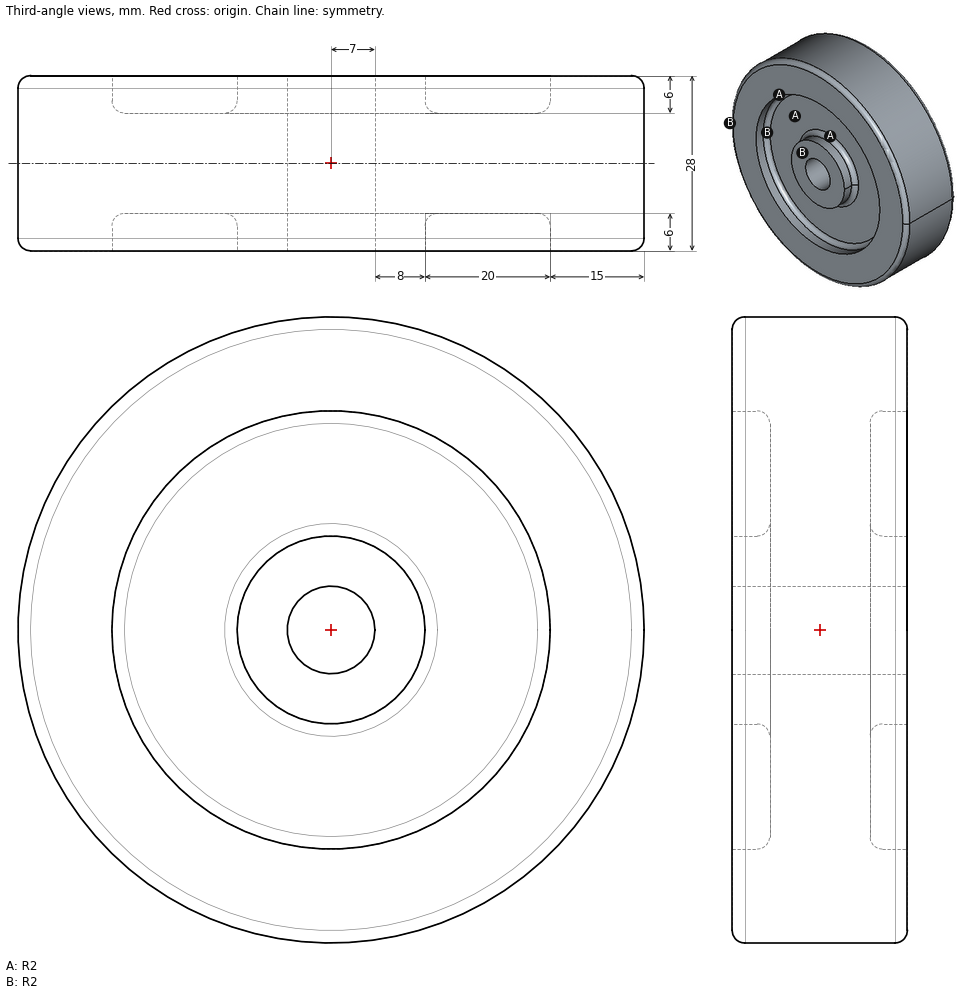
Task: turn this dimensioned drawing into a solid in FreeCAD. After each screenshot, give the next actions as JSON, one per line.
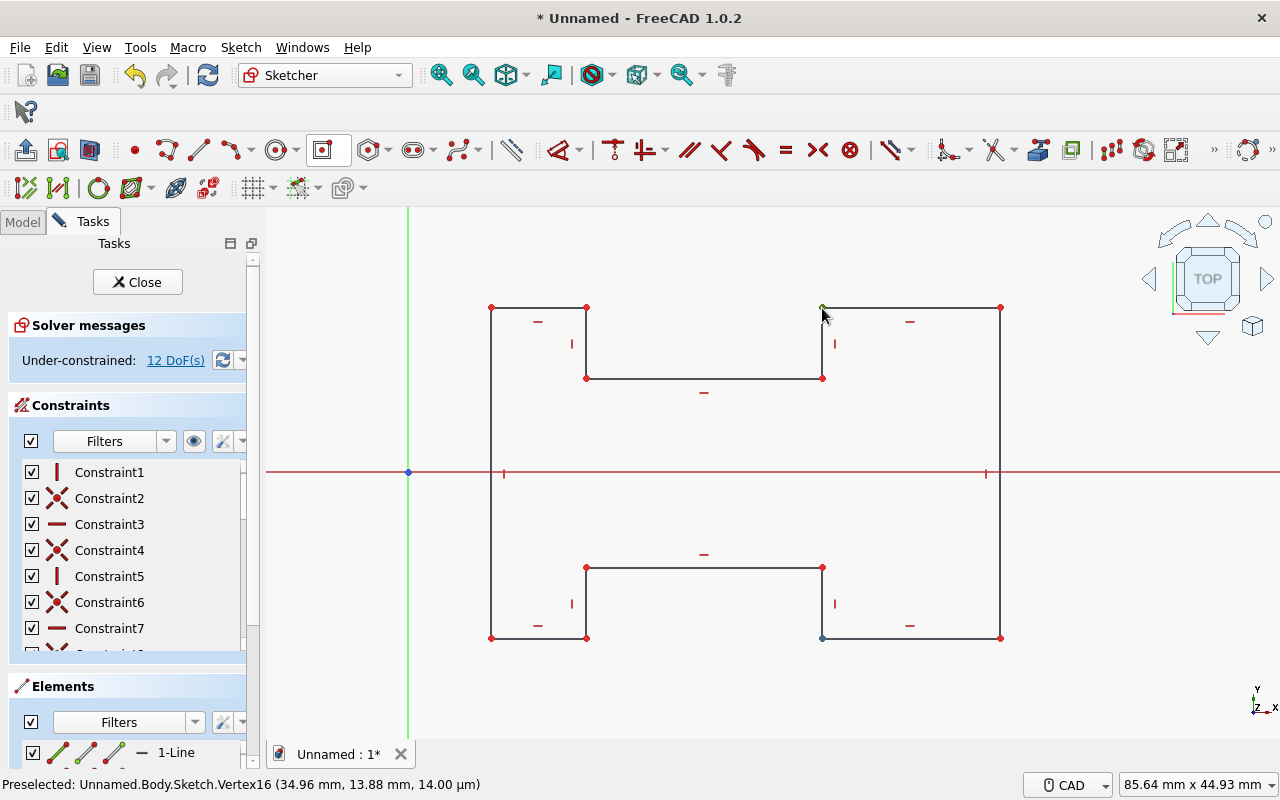
{"action": "left_click", "coordinate": [353, 472]}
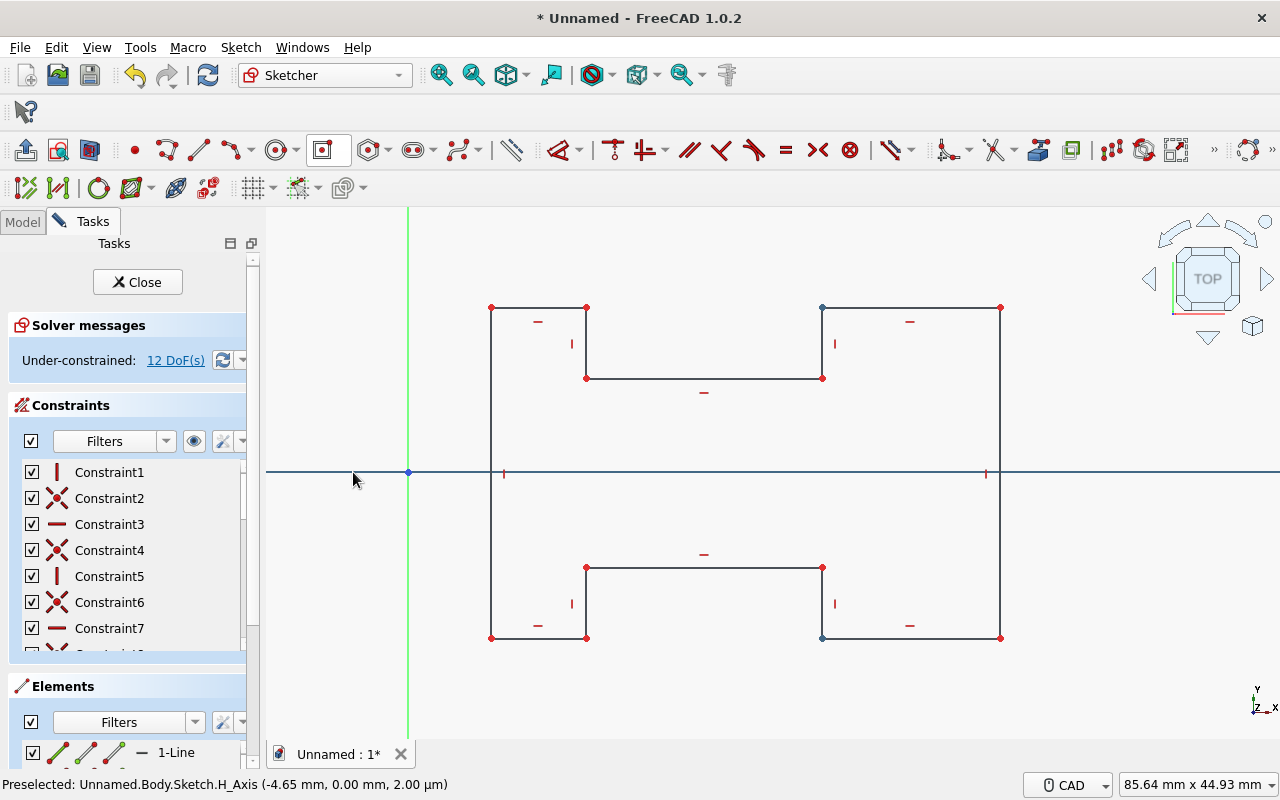
{"action": "left_click", "coordinate": [818, 150]}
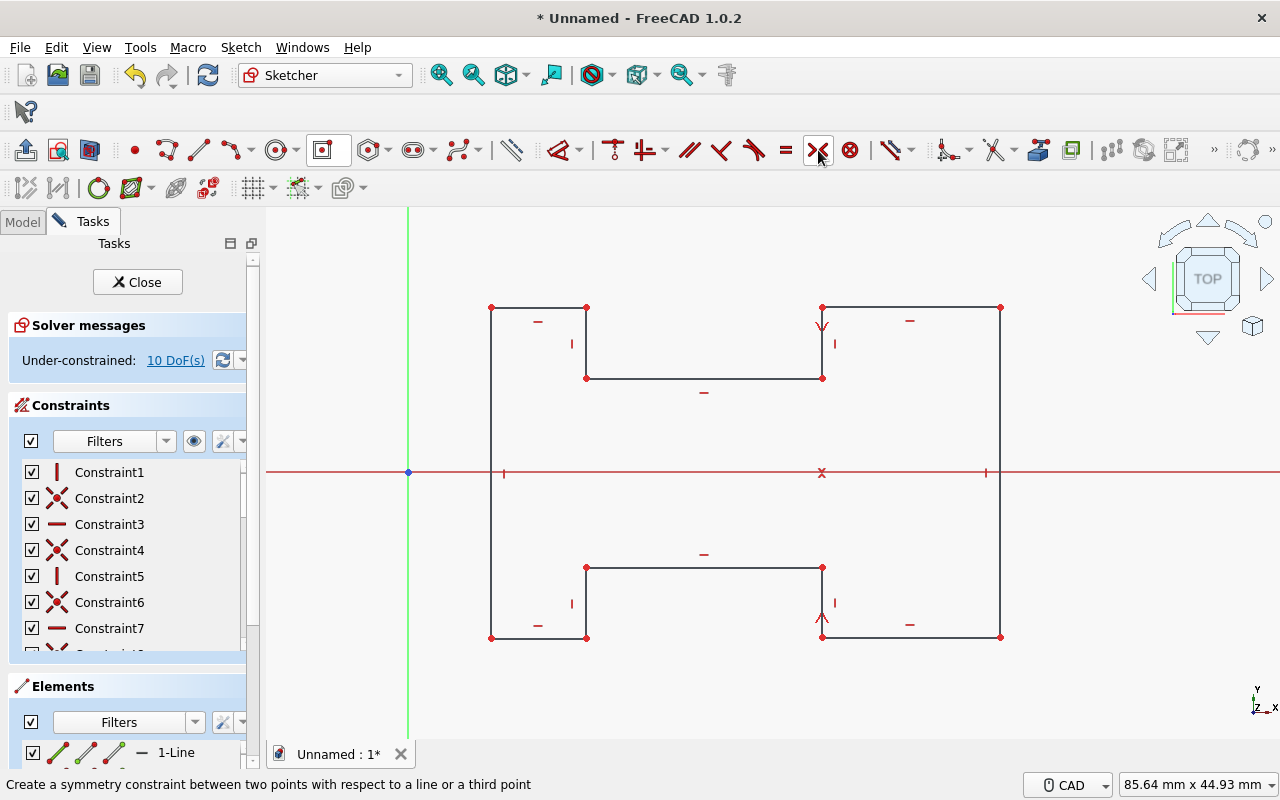
{"action": "left_click", "coordinate": [586, 568]}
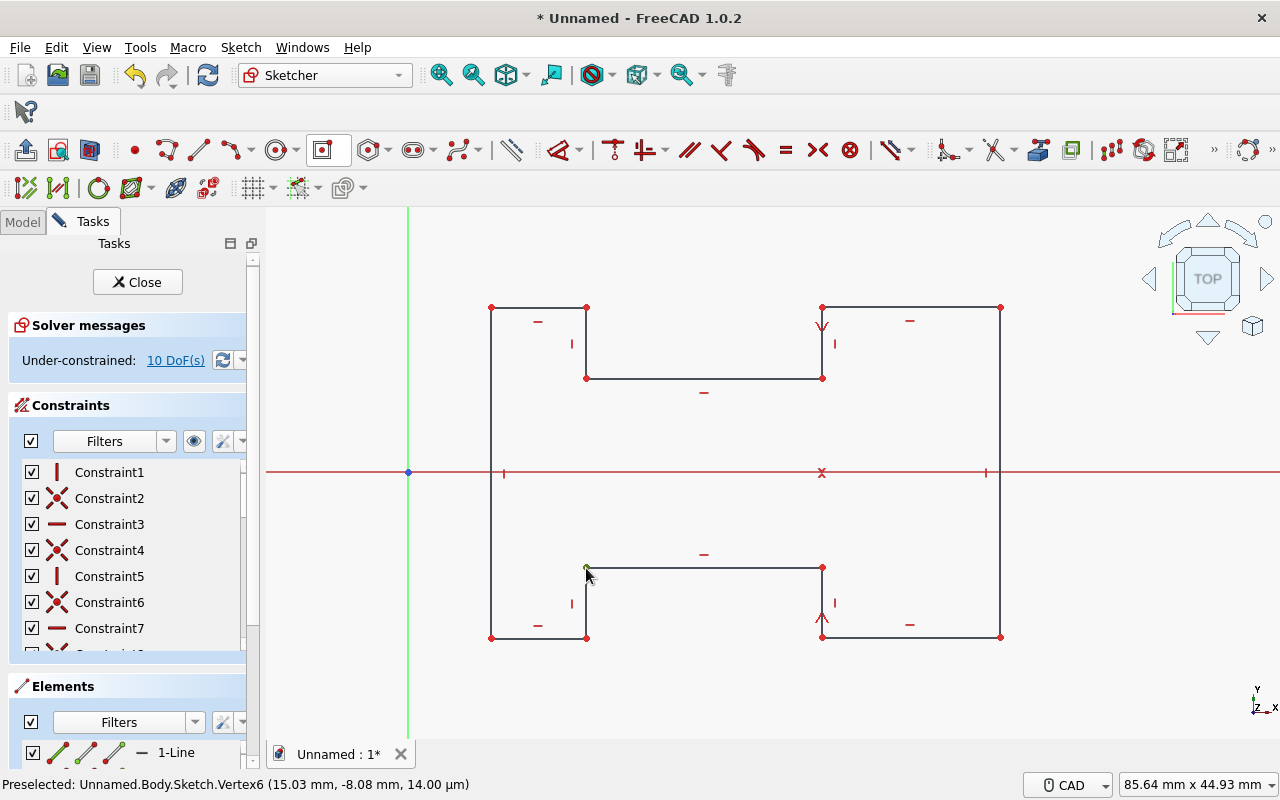
{"action": "left_click", "coordinate": [586, 379]}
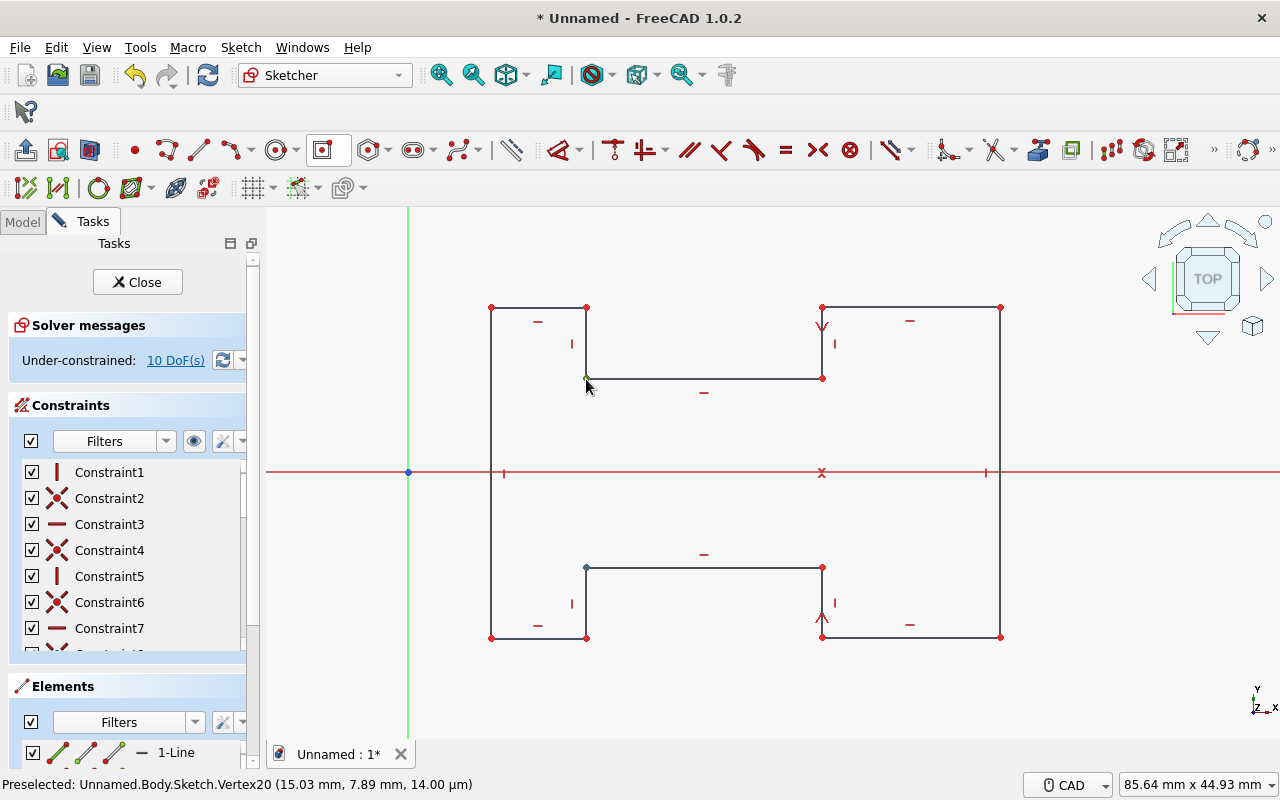
{"action": "left_click", "coordinate": [353, 472]}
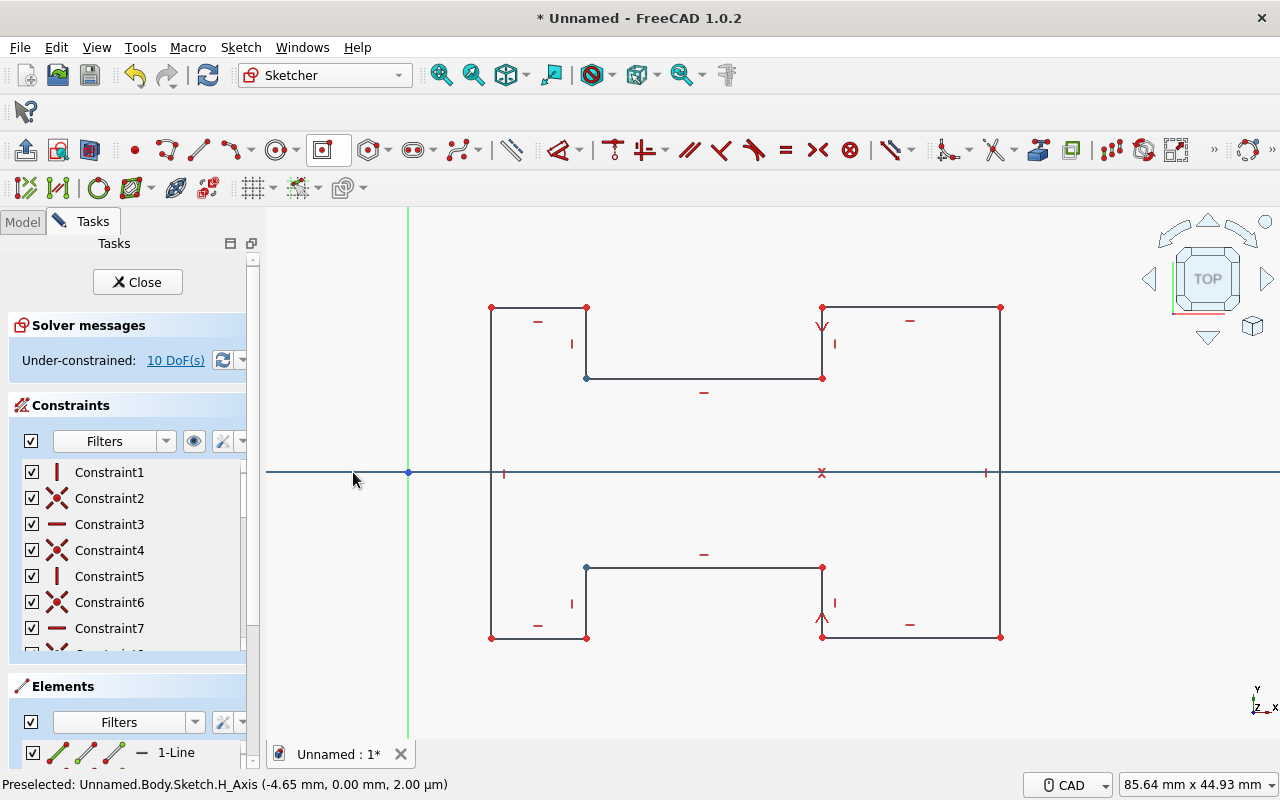
{"action": "left_click", "coordinate": [818, 150]}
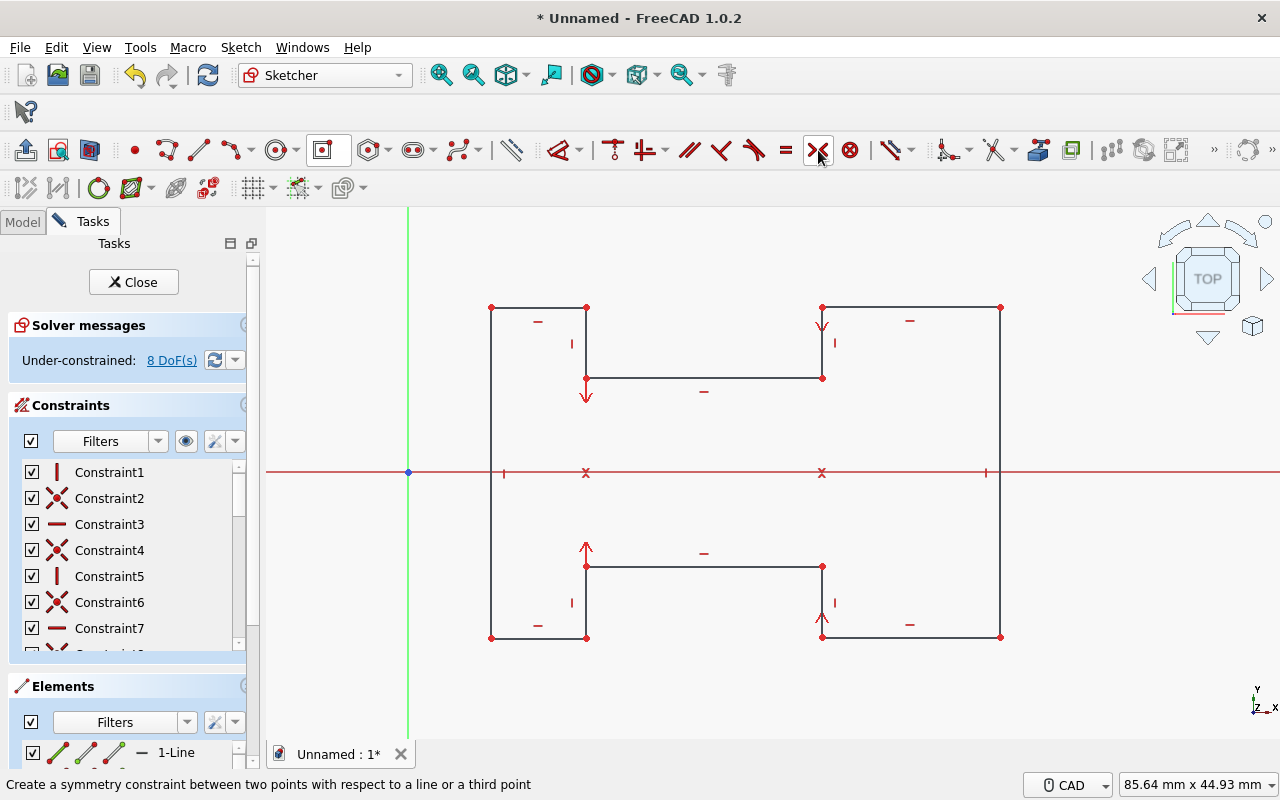
{"action": "left_click", "coordinate": [558, 150]}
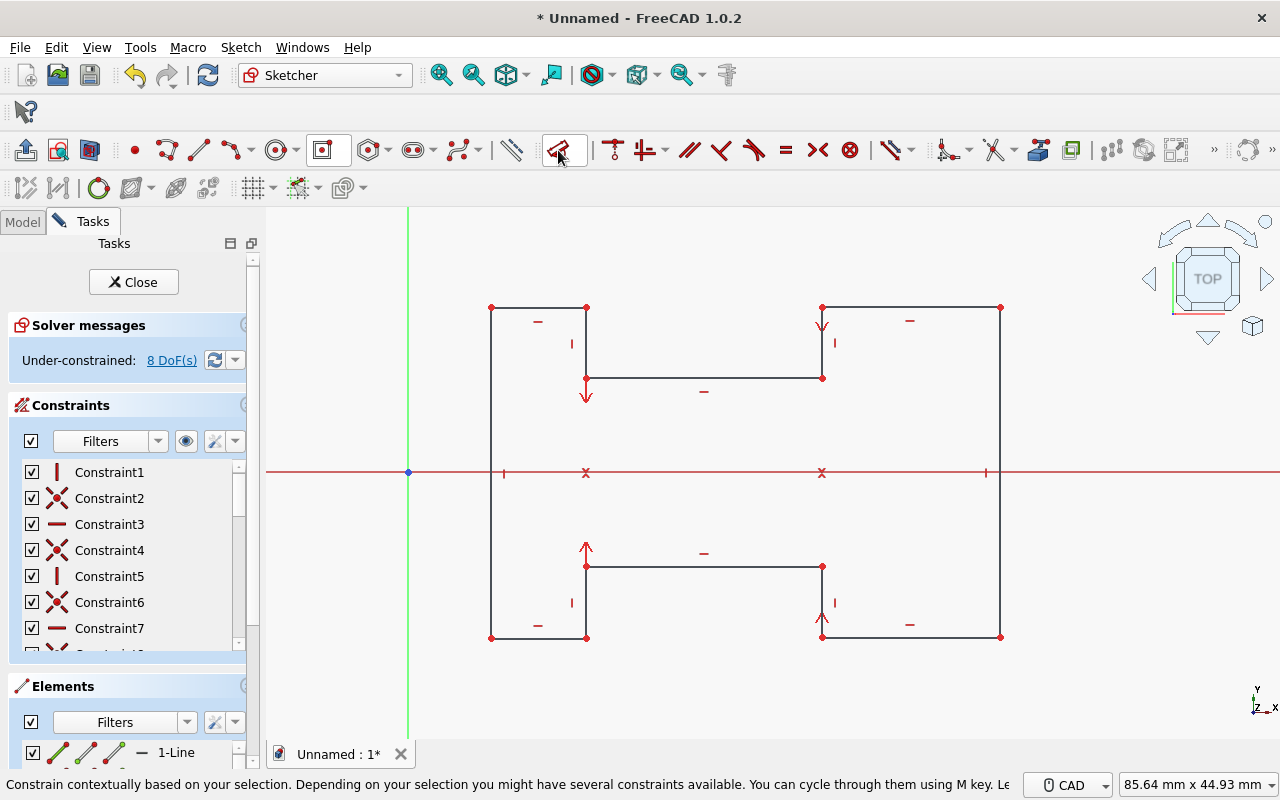
{"action": "left_click", "coordinate": [519, 639]}
{"action": "left_click", "coordinate": [538, 673]}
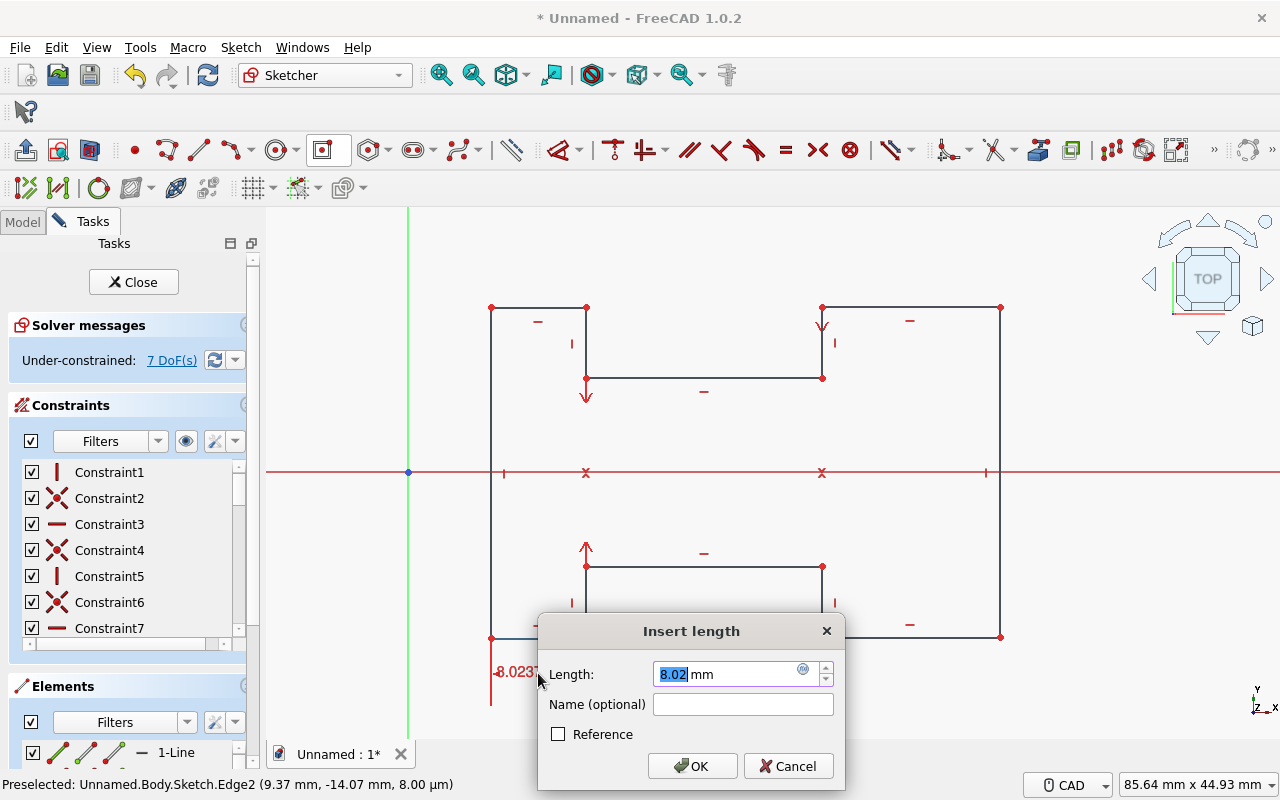
{"action": "type", "text": "8"}
{"action": "key", "text": "Return"}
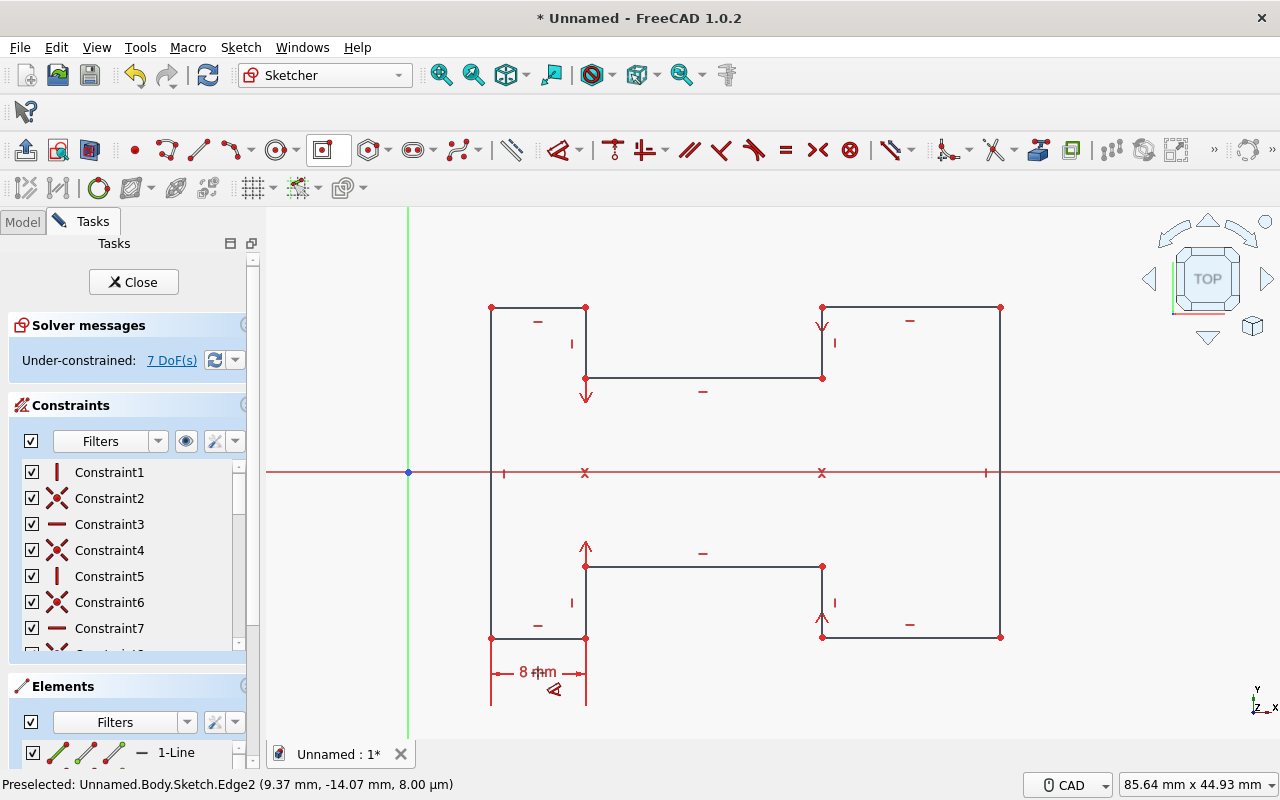
{"action": "left_click", "coordinate": [586, 617]}
{"action": "left_click", "coordinate": [552, 603]}